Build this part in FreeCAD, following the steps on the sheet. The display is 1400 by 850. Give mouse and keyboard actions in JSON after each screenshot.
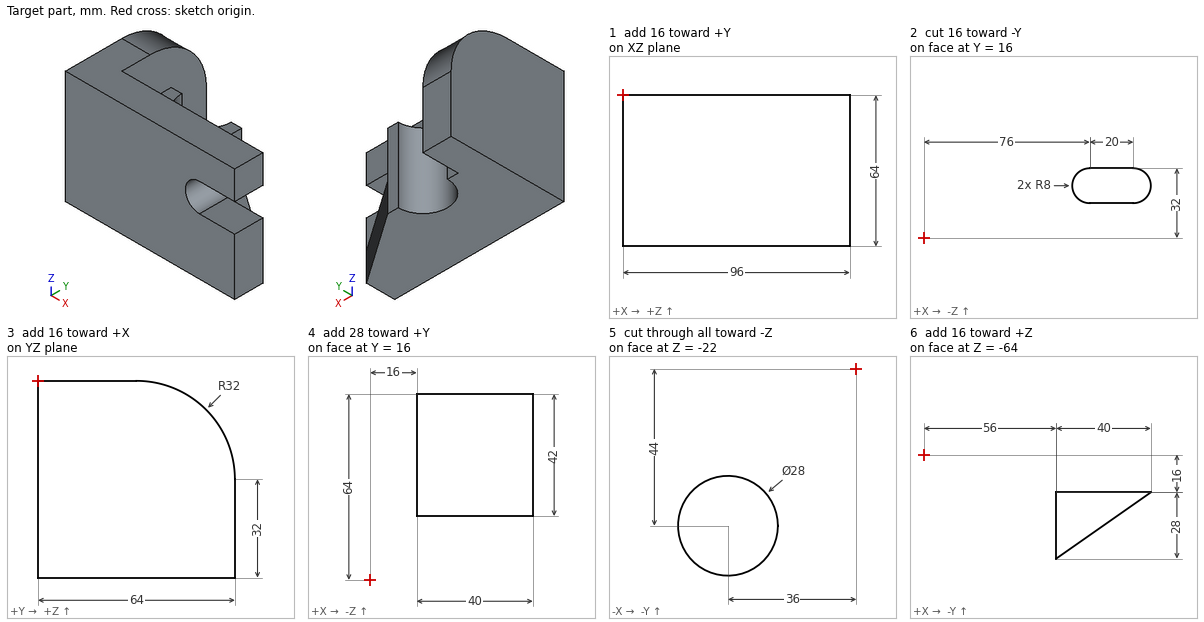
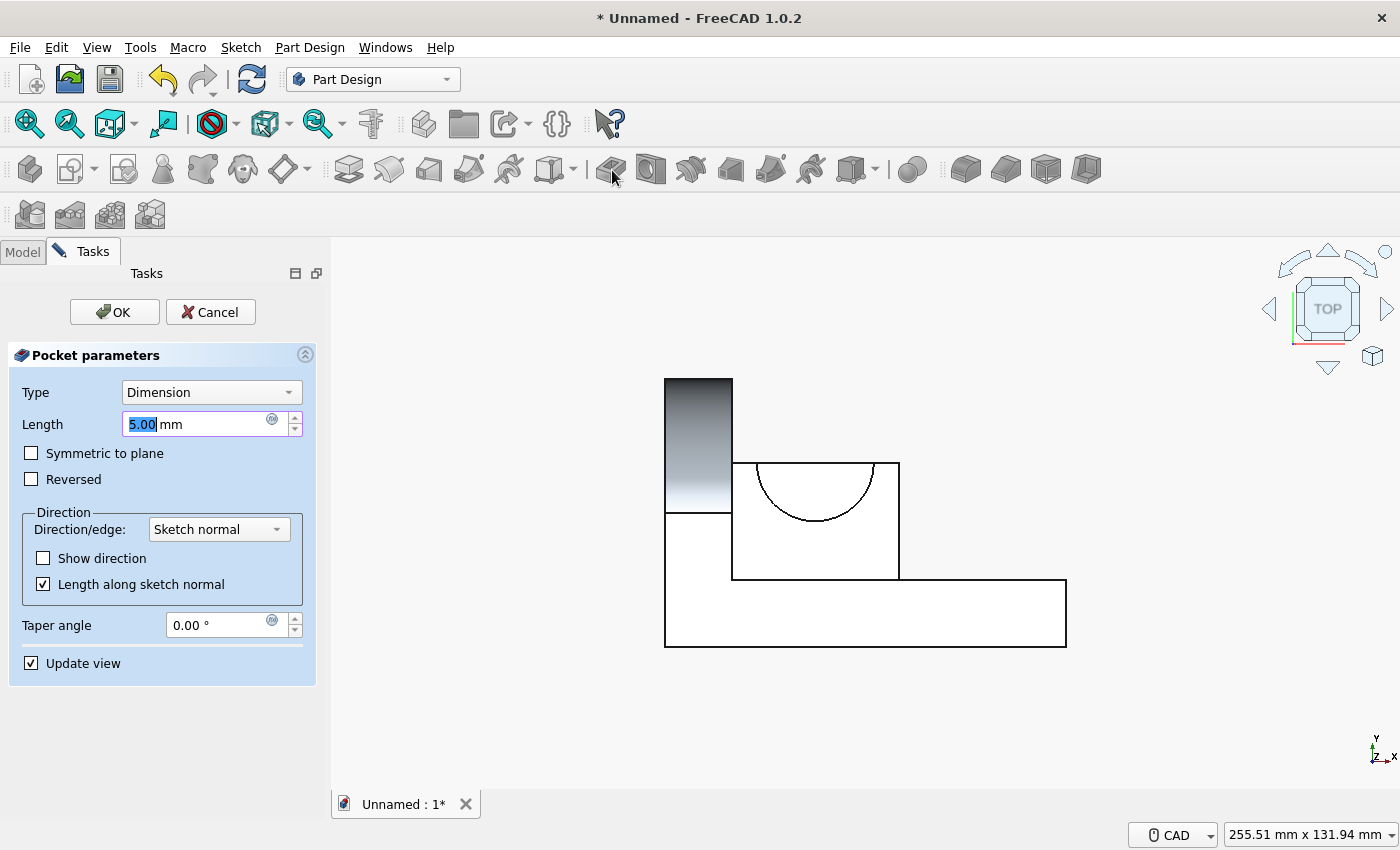
{"action": "left_click", "coordinate": [212, 392]}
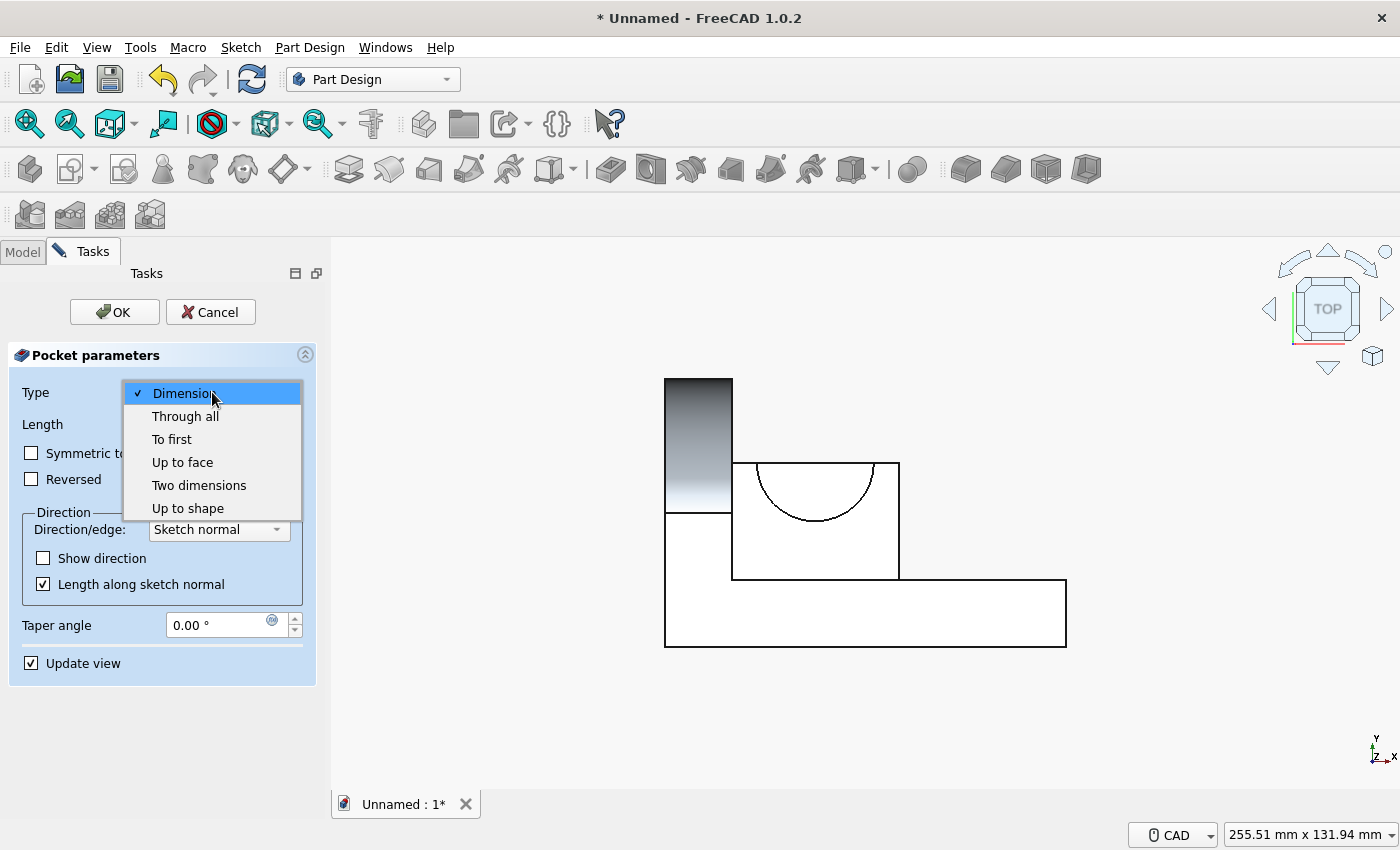
{"action": "left_click", "coordinate": [212, 416]}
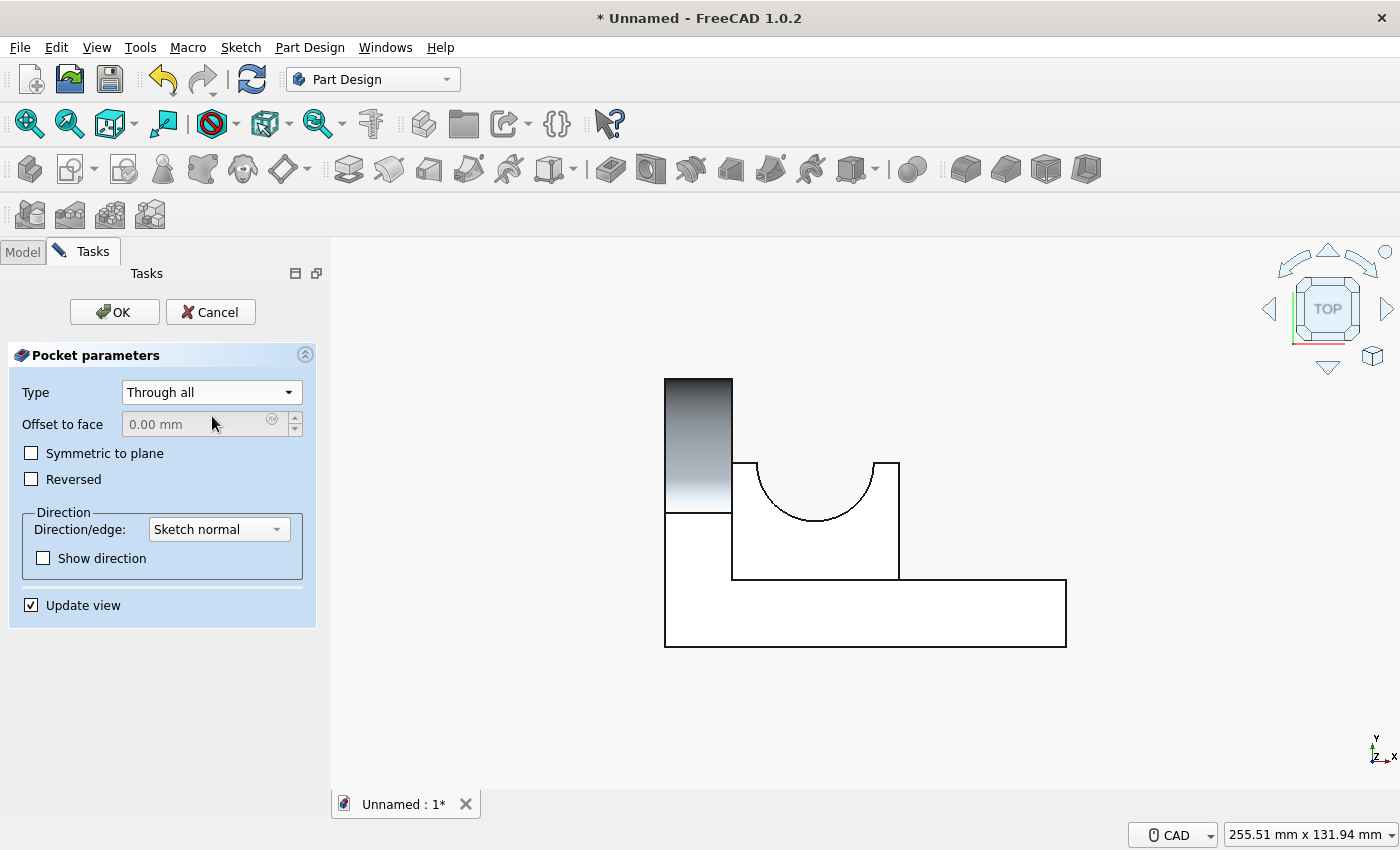
{"action": "left_click", "coordinate": [115, 312]}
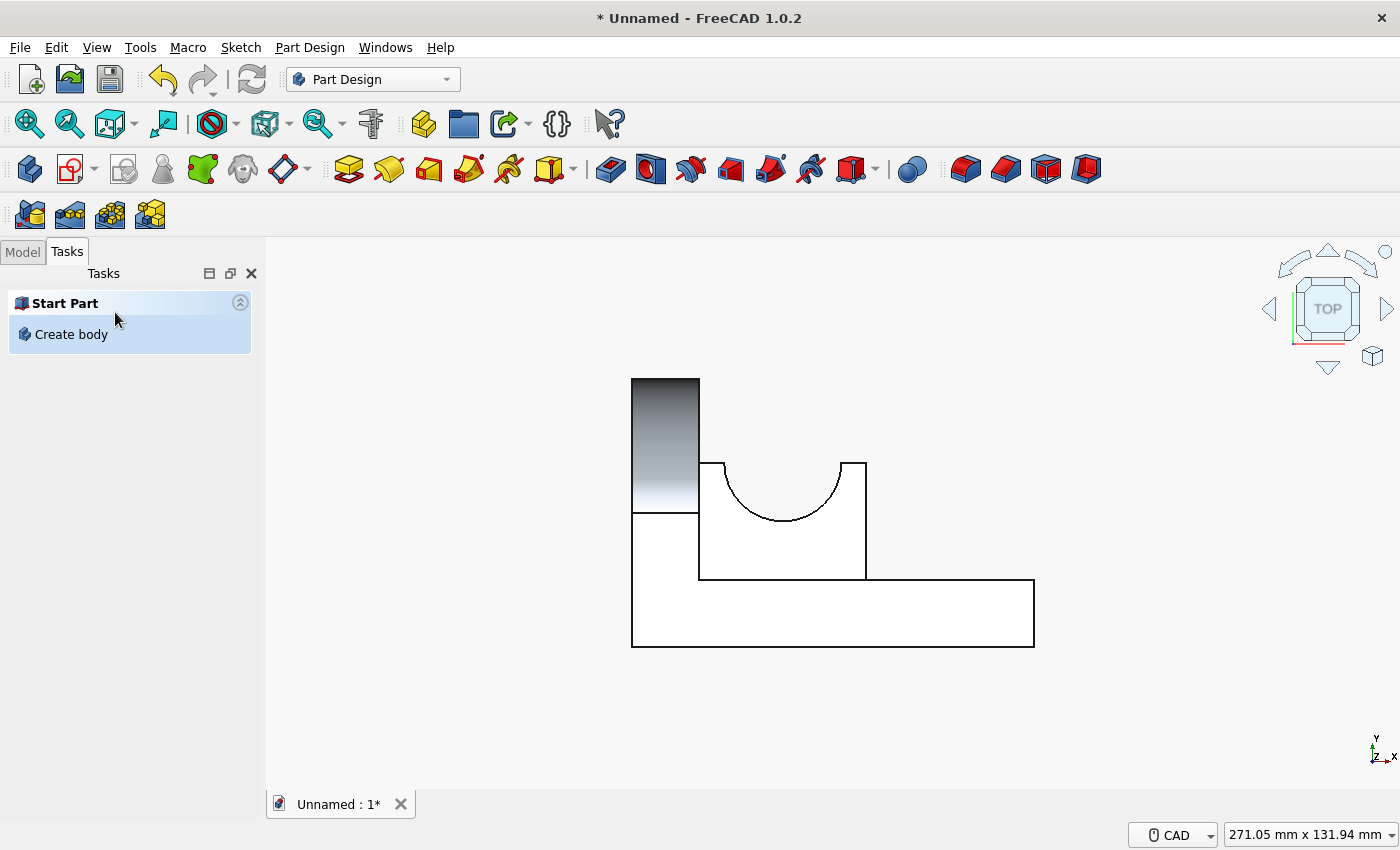
{"action": "key", "text": "5"}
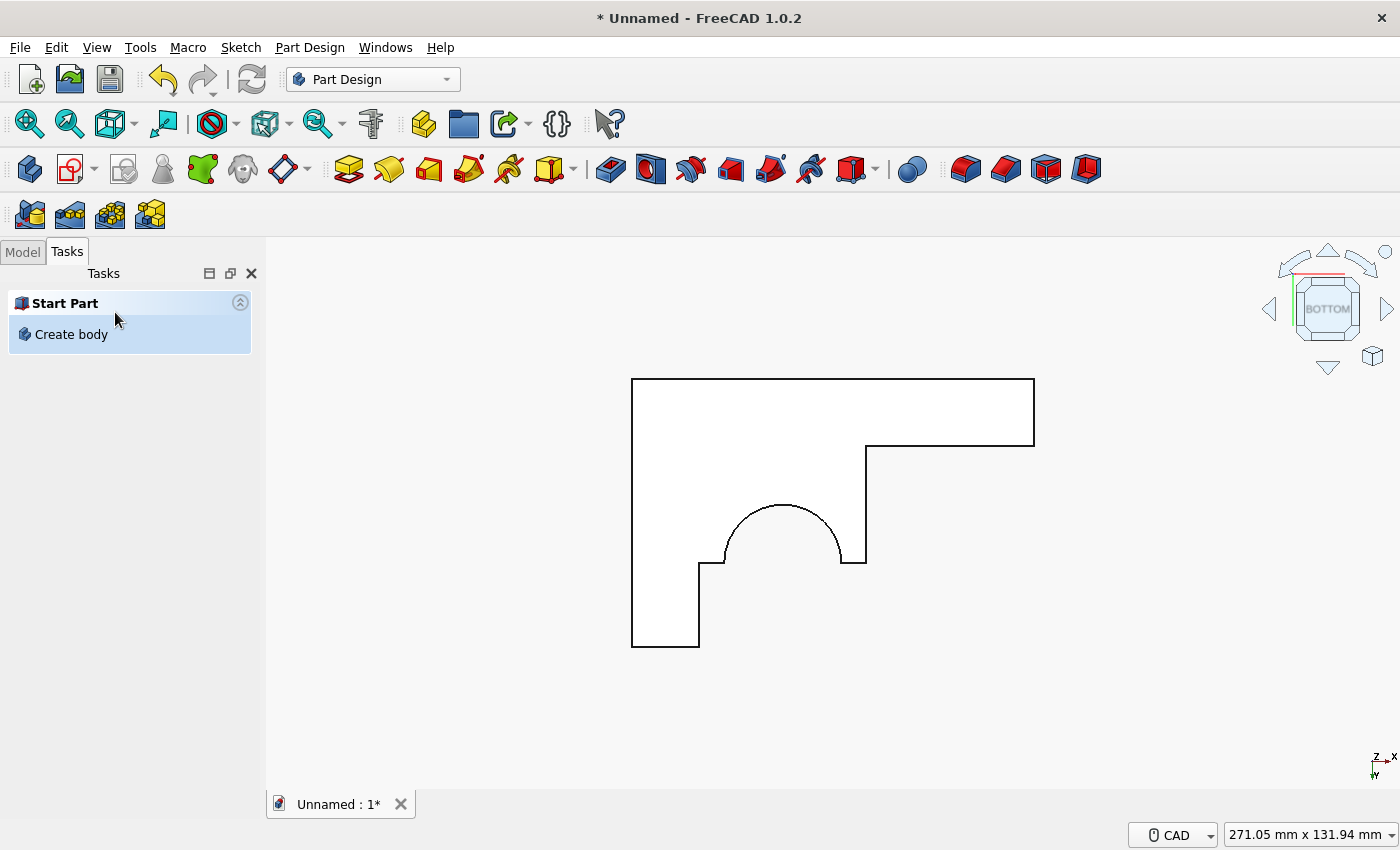
{"action": "left_click", "coordinate": [776, 435]}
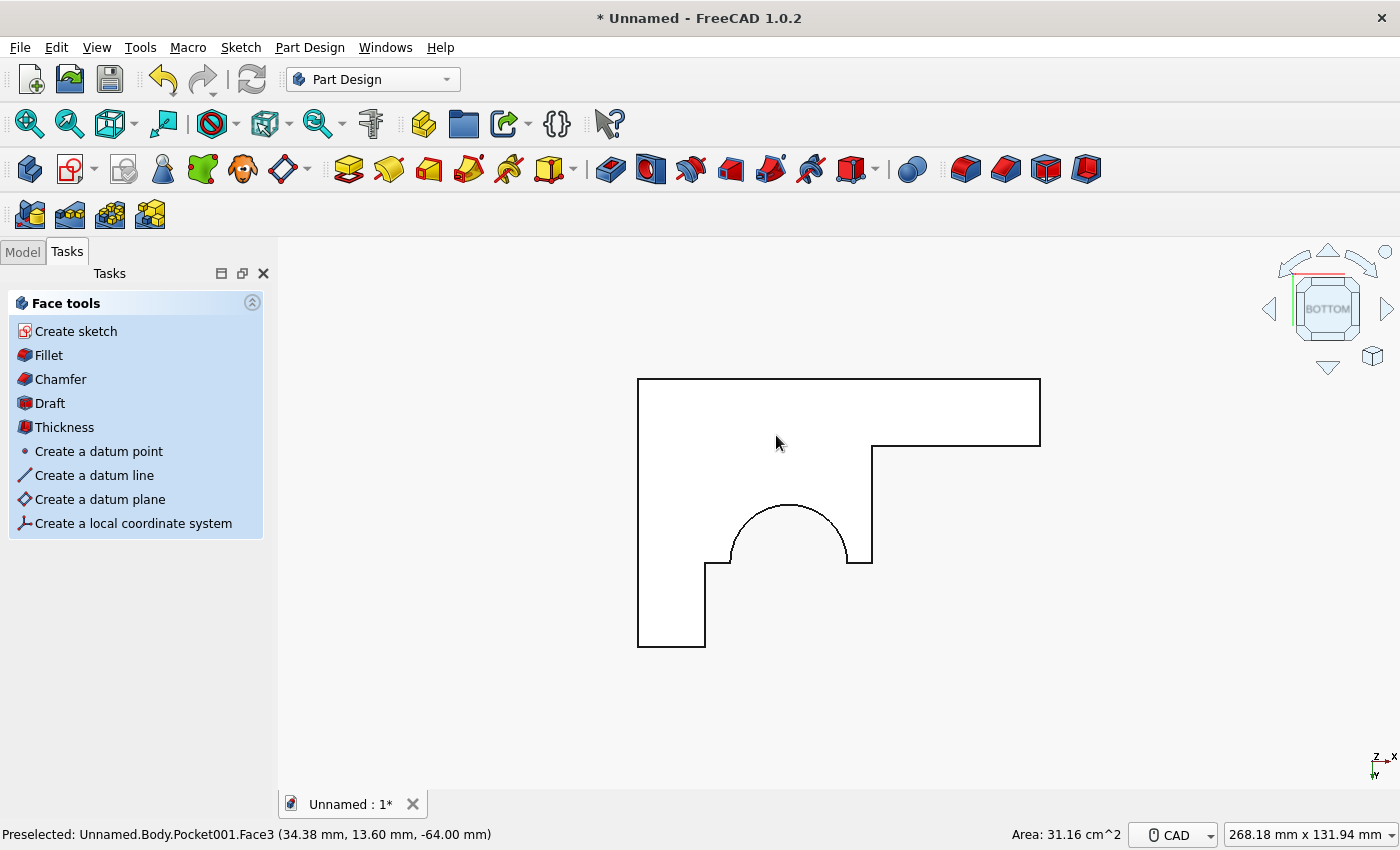
{"action": "left_click", "coordinate": [70, 170]}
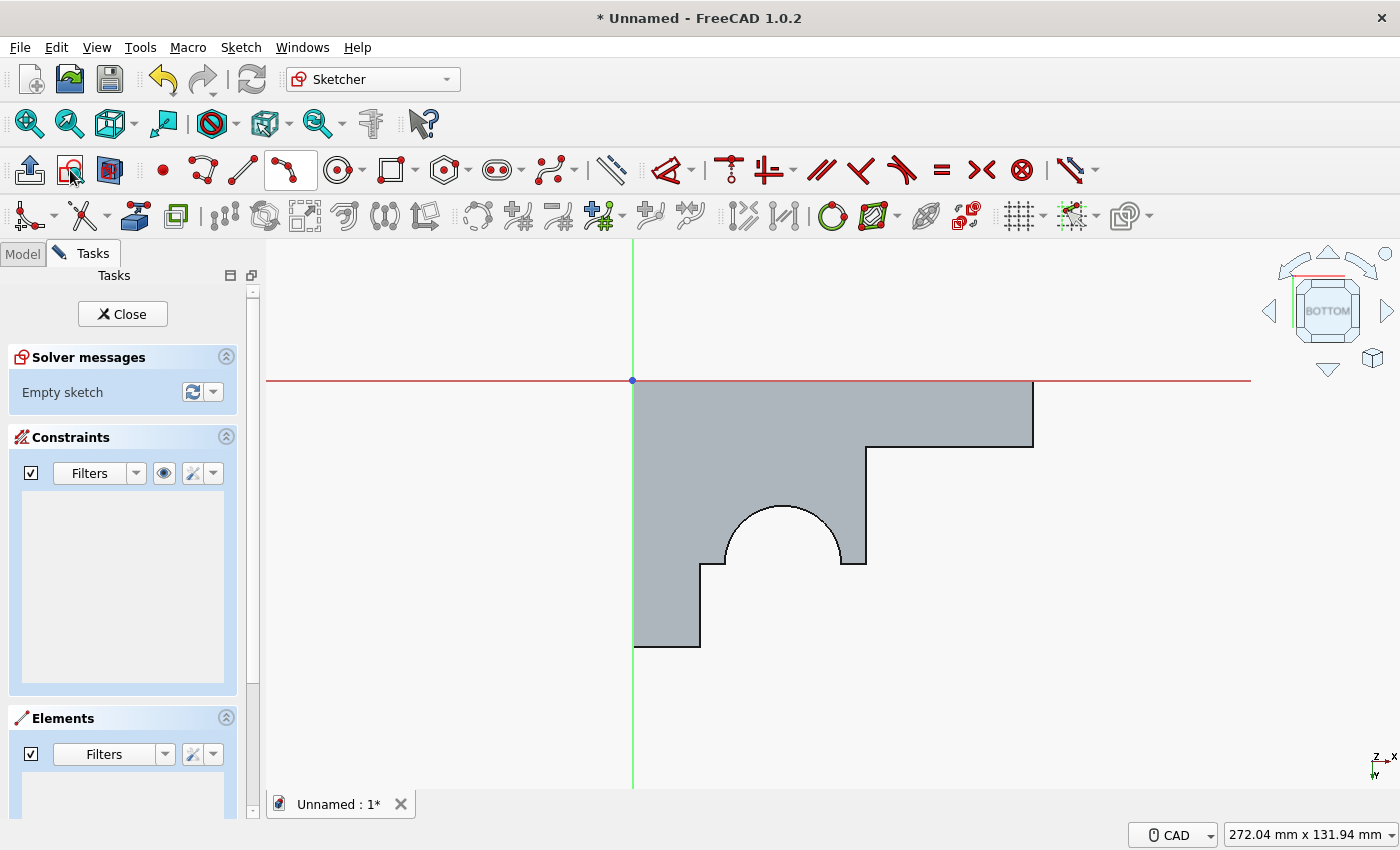
{"action": "scroll", "coordinate": [916, 422], "scroll_direction": "up", "scroll_amount": 3}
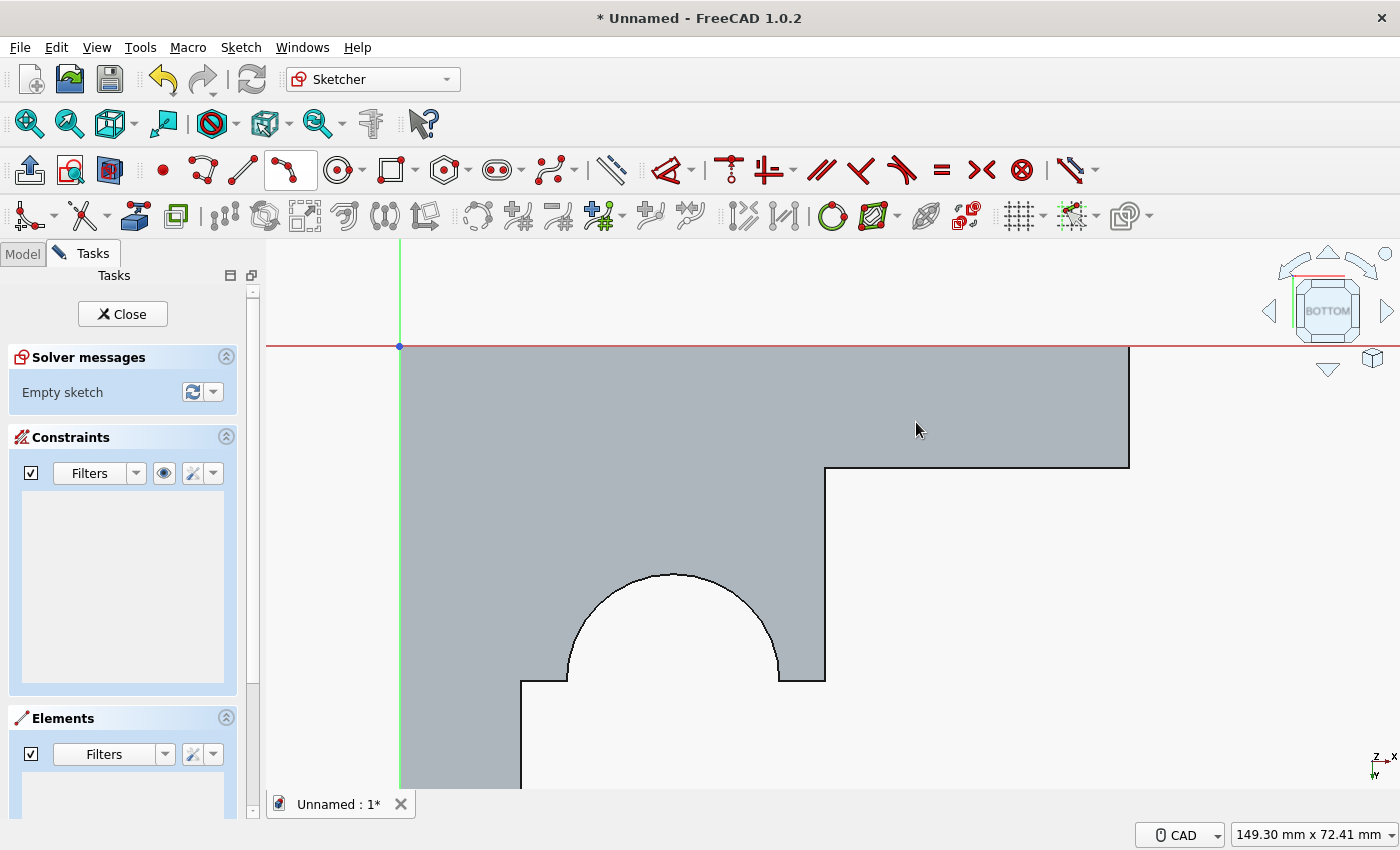
{"action": "left_click", "coordinate": [204, 170]}